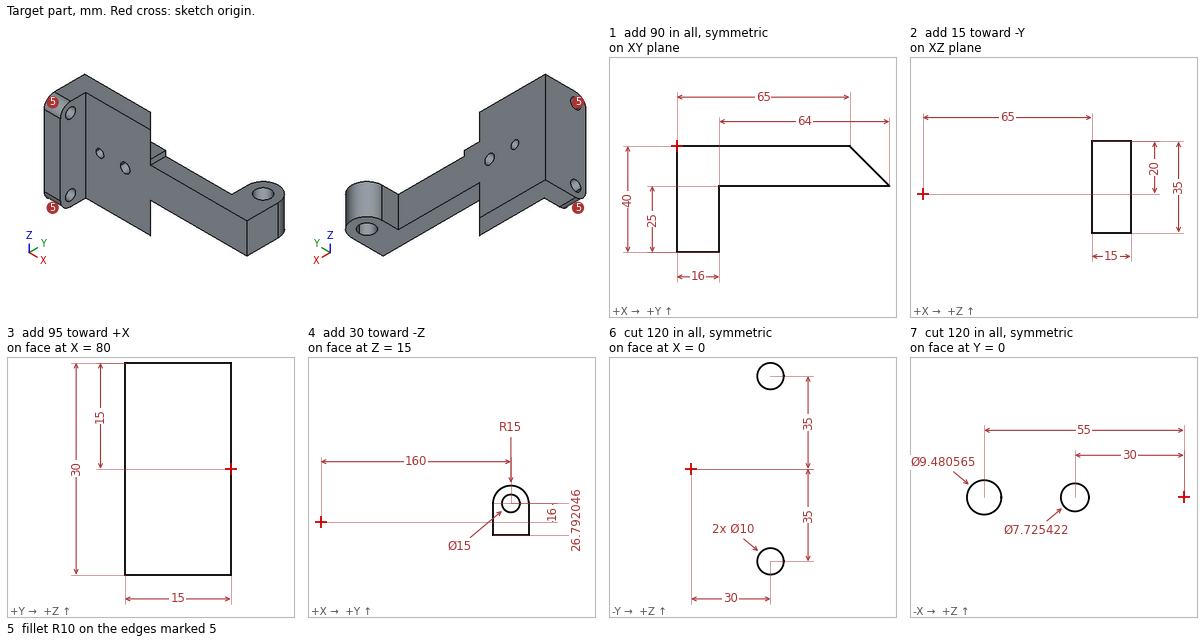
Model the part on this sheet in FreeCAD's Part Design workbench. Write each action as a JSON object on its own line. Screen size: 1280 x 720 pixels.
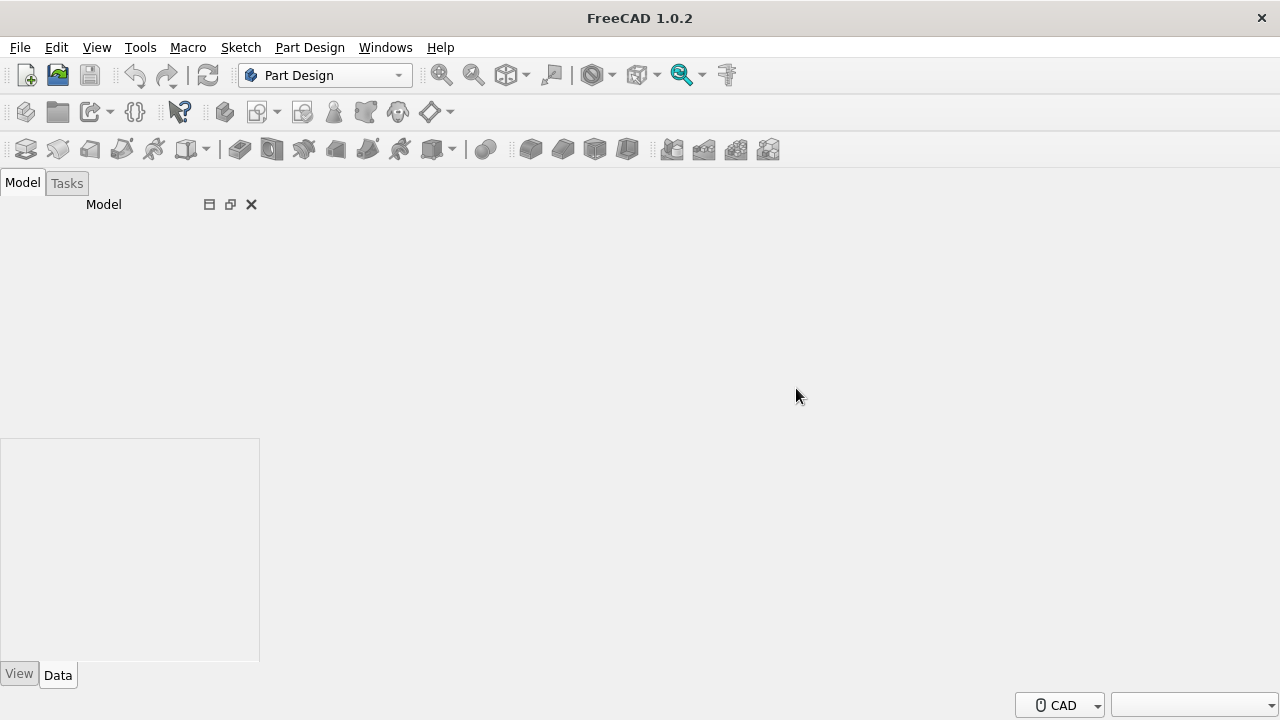
{"action": "left_click", "coordinate": [26, 76]}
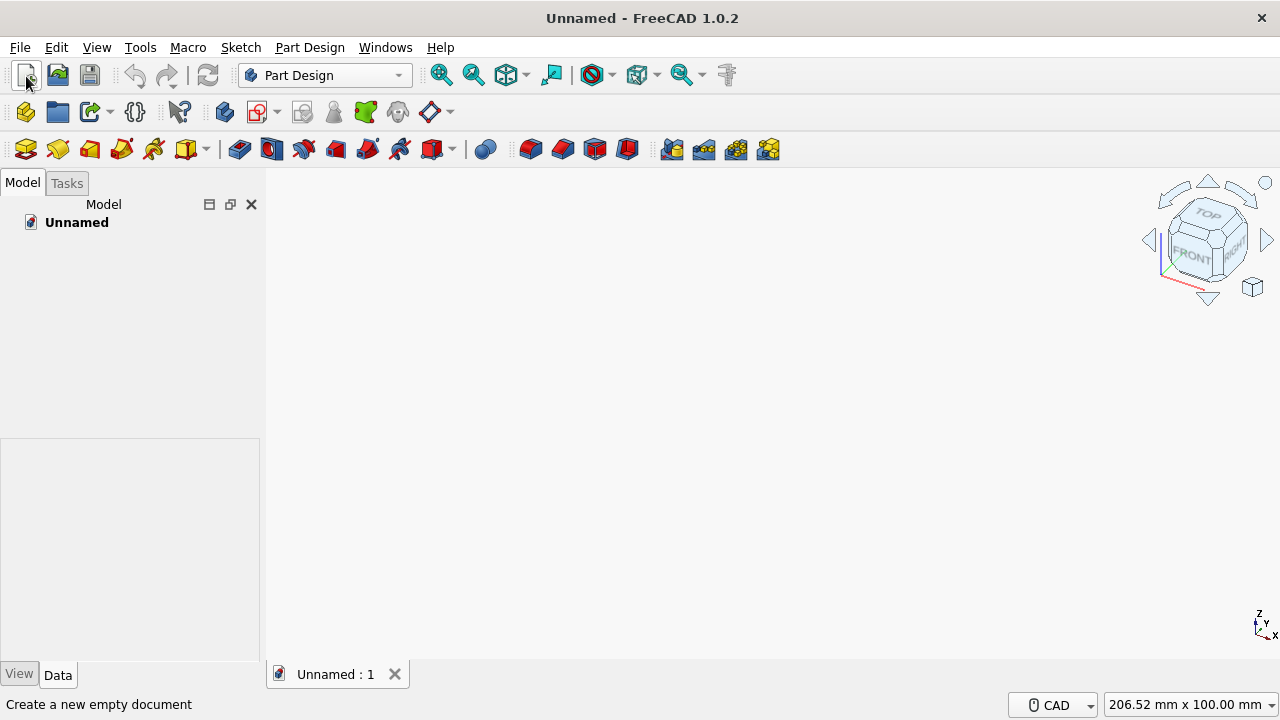
{"action": "left_click", "coordinate": [258, 112]}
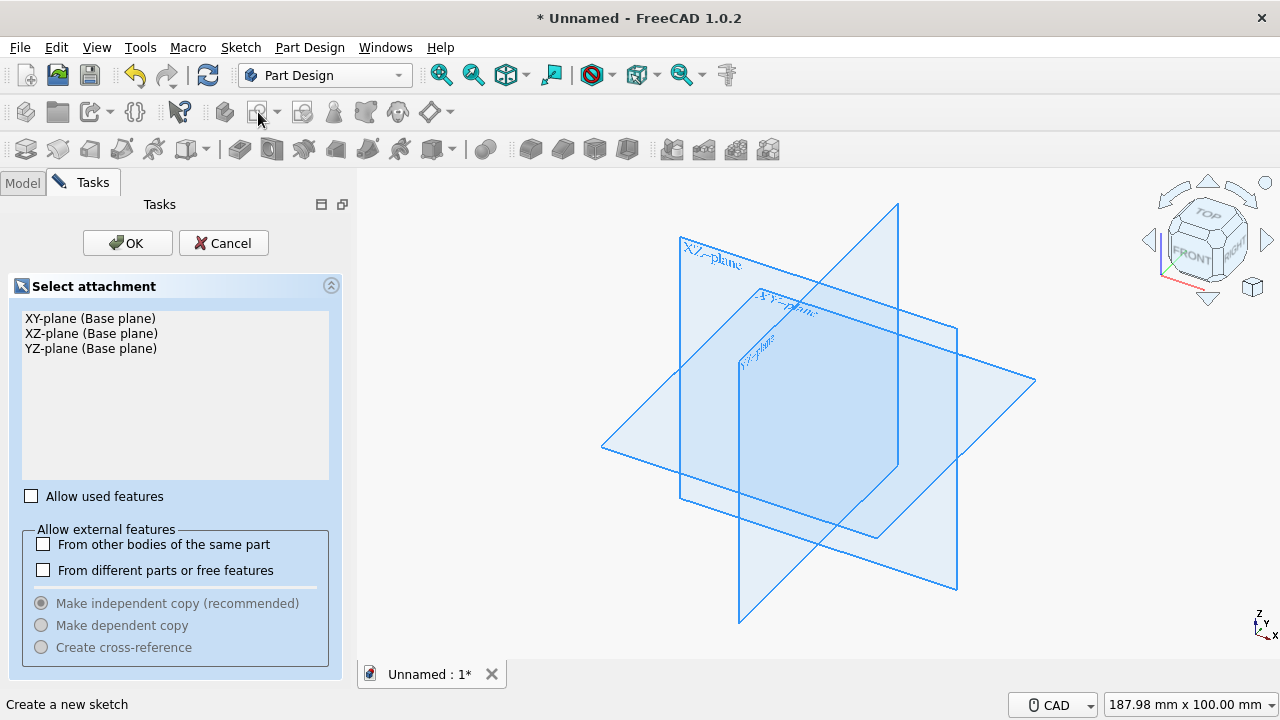
{"action": "left_click", "coordinate": [82, 318]}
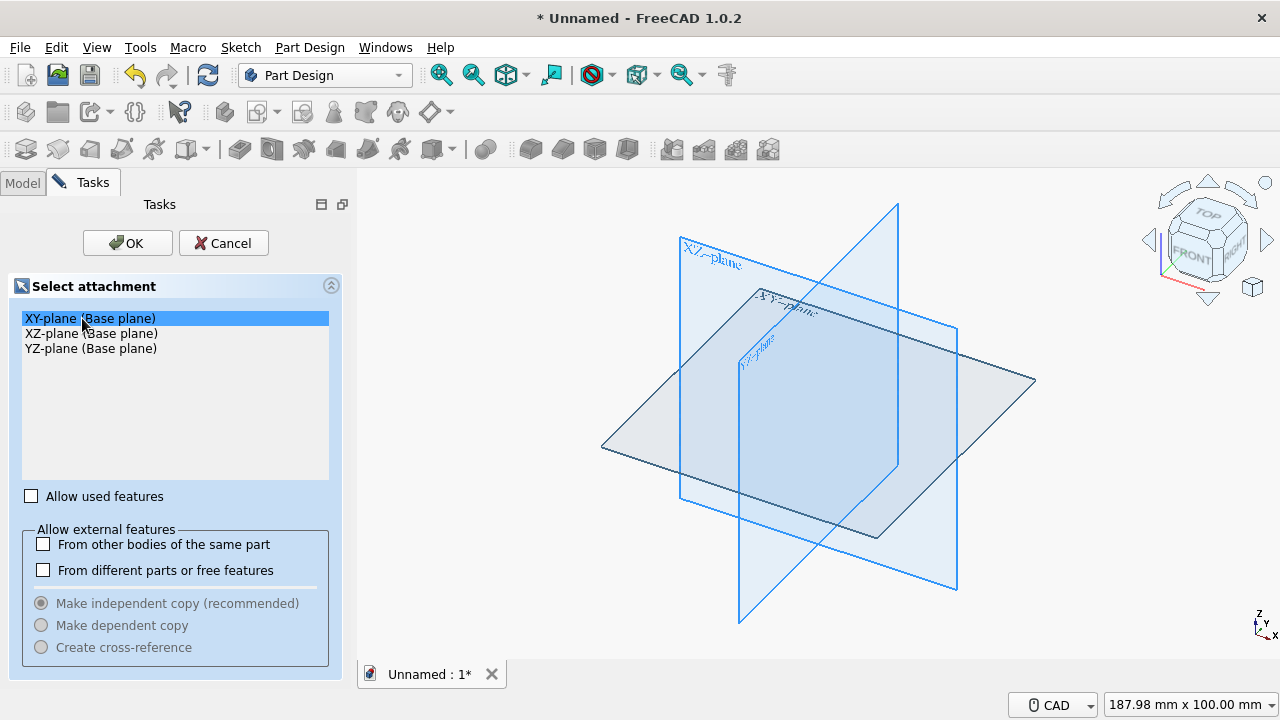
{"action": "left_click", "coordinate": [128, 243]}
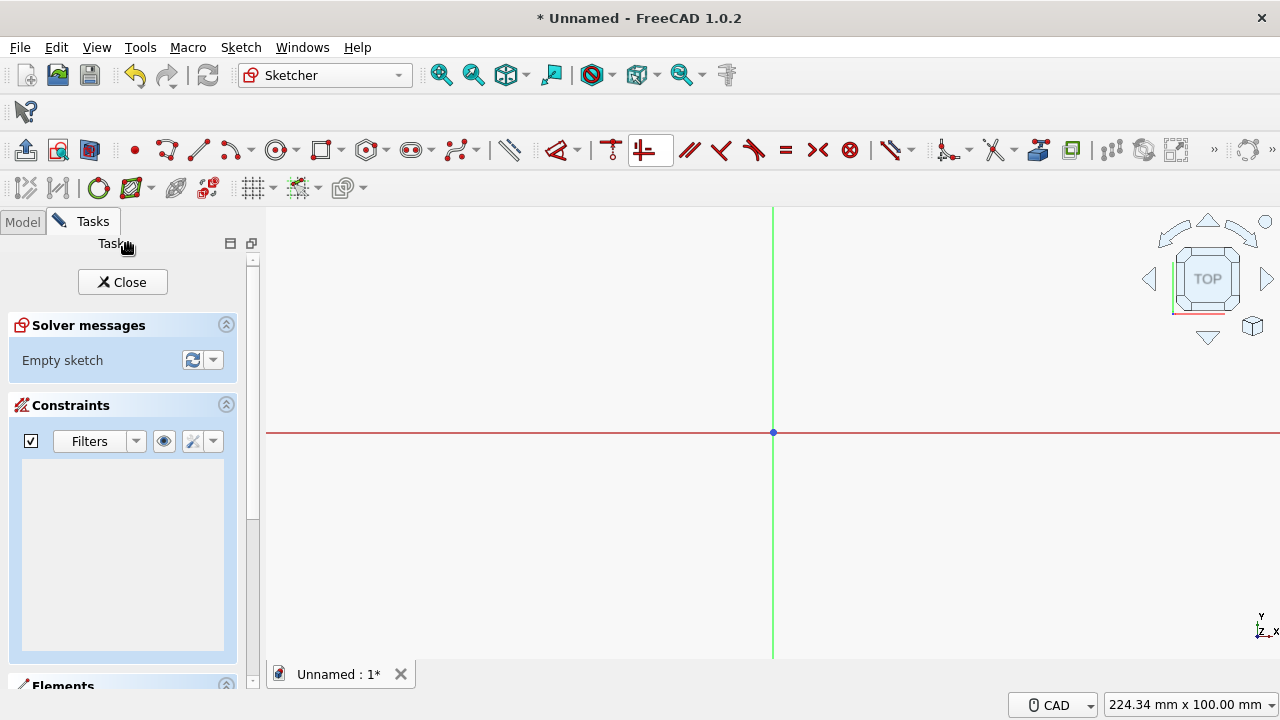
{"action": "scroll", "coordinate": [294, 235], "scroll_direction": "down", "scroll_amount": 1}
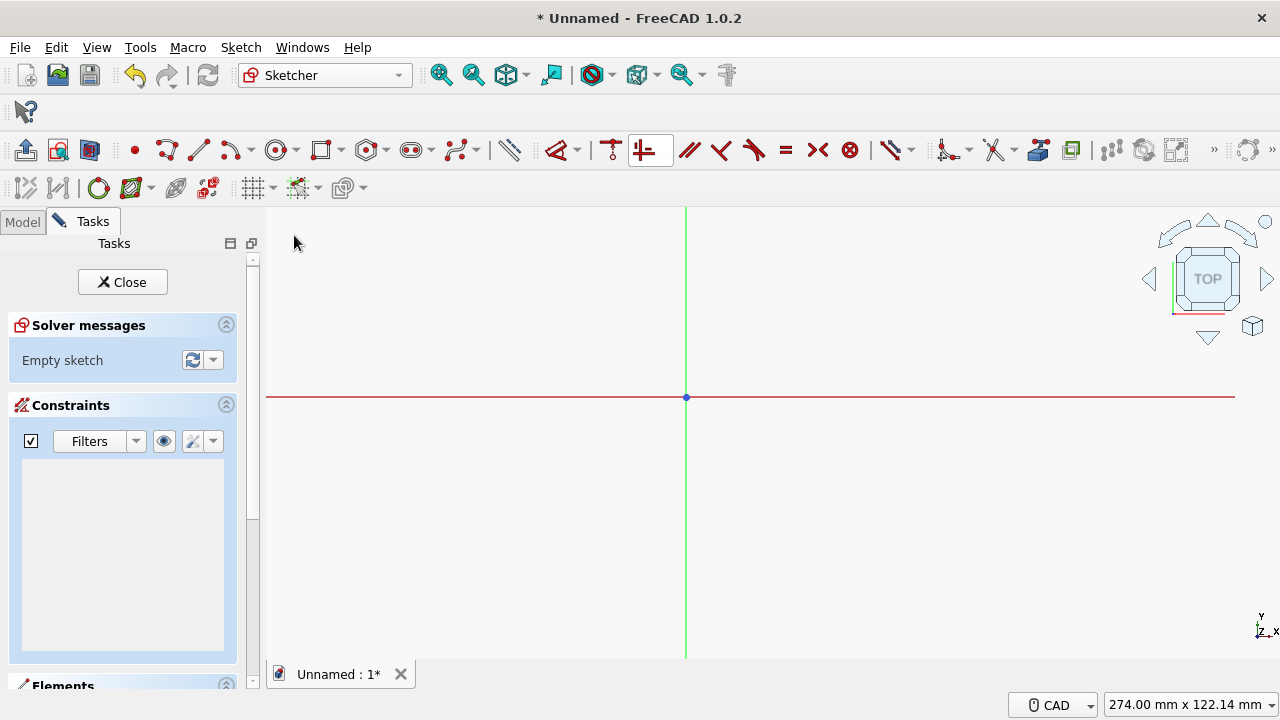
{"action": "scroll", "coordinate": [992, 518], "scroll_direction": "up", "scroll_amount": 3}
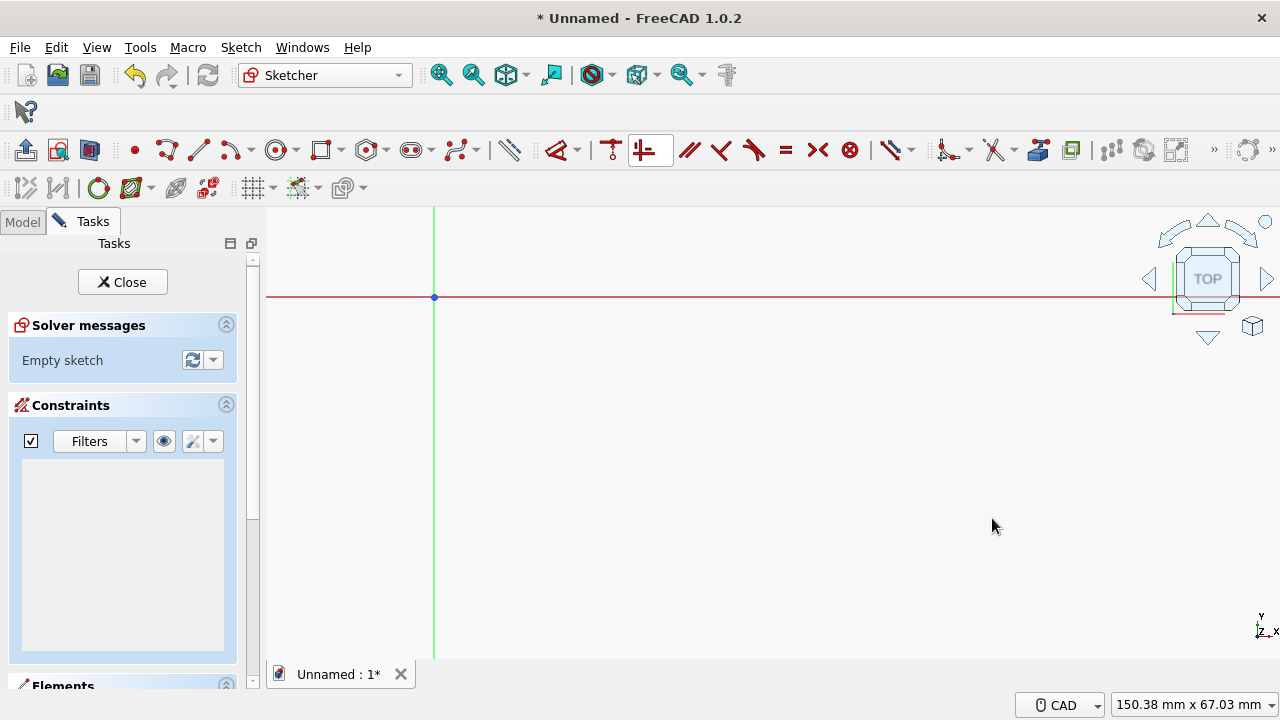
{"action": "left_click", "coordinate": [168, 150]}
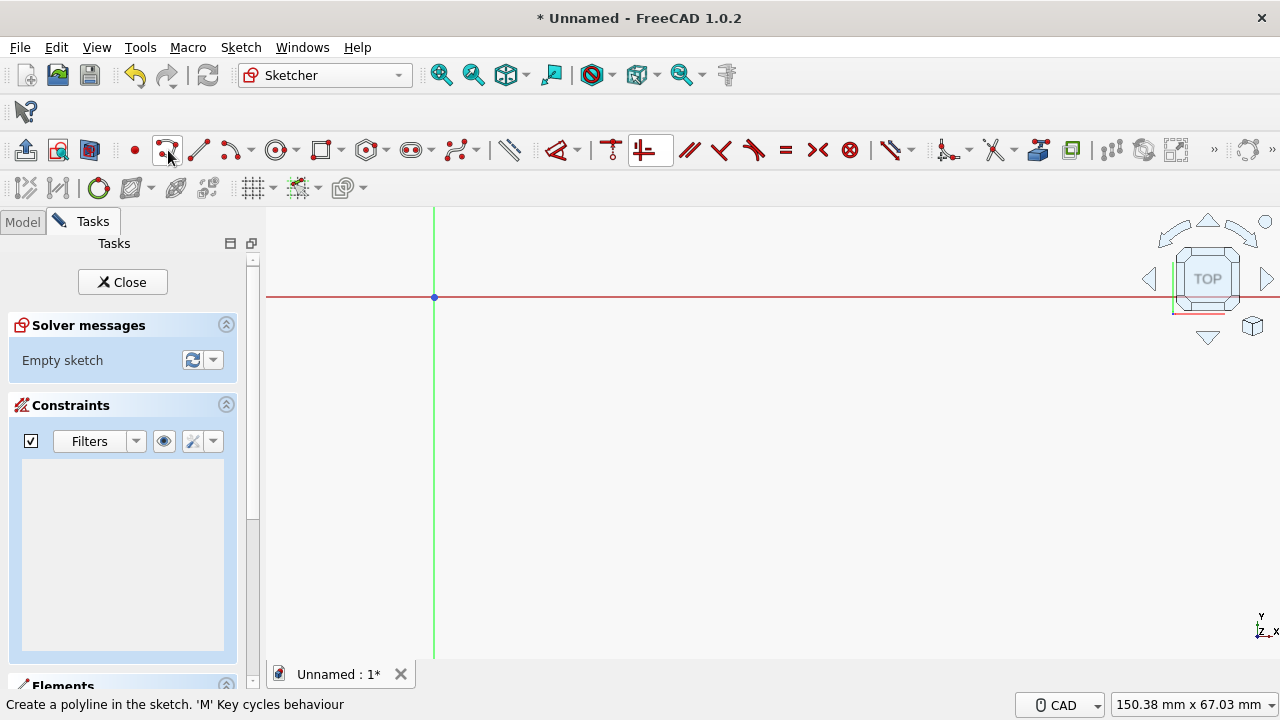
{"action": "left_click", "coordinate": [434, 297]}
{"action": "left_click", "coordinate": [443, 567]}
{"action": "left_click", "coordinate": [542, 567]}
{"action": "left_click", "coordinate": [542, 398]}
{"action": "left_click", "coordinate": [974, 398]}
{"action": "left_click", "coordinate": [872, 306]}
{"action": "left_click", "coordinate": [434, 297]}
{"action": "key", "text": "Escape"}
{"action": "key", "text": "Escape"}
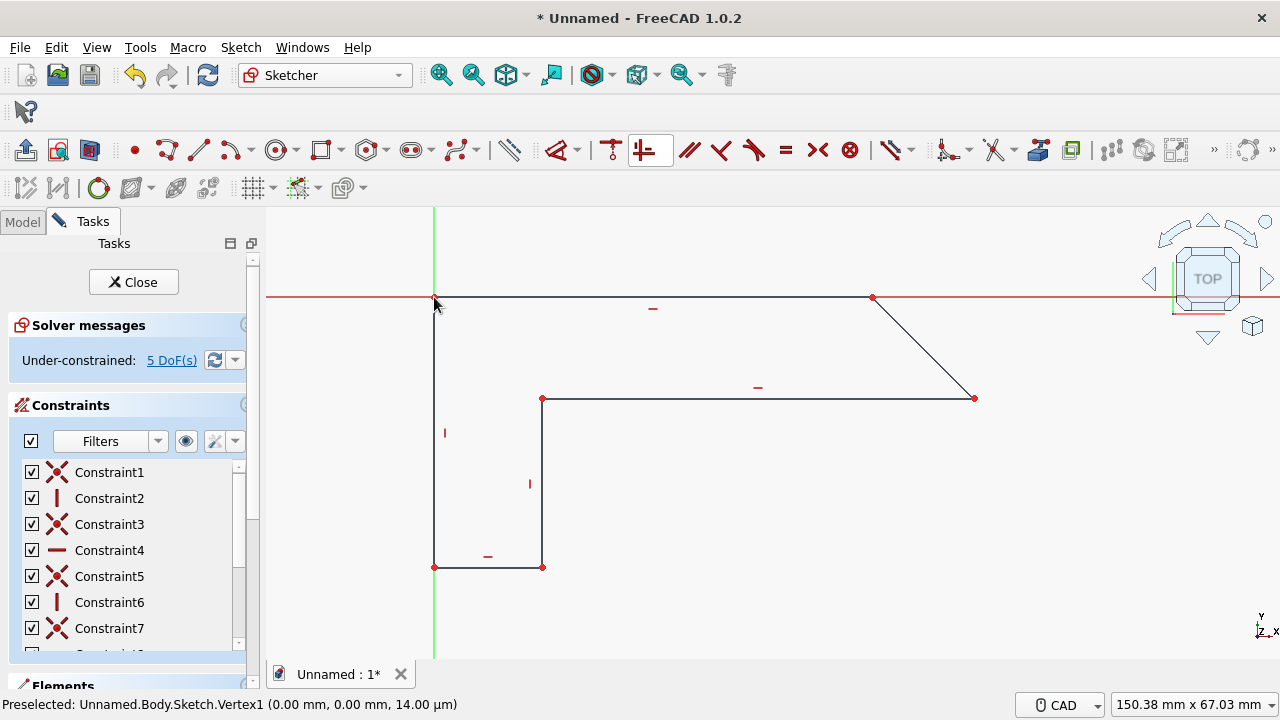
{"action": "left_click", "coordinate": [556, 150]}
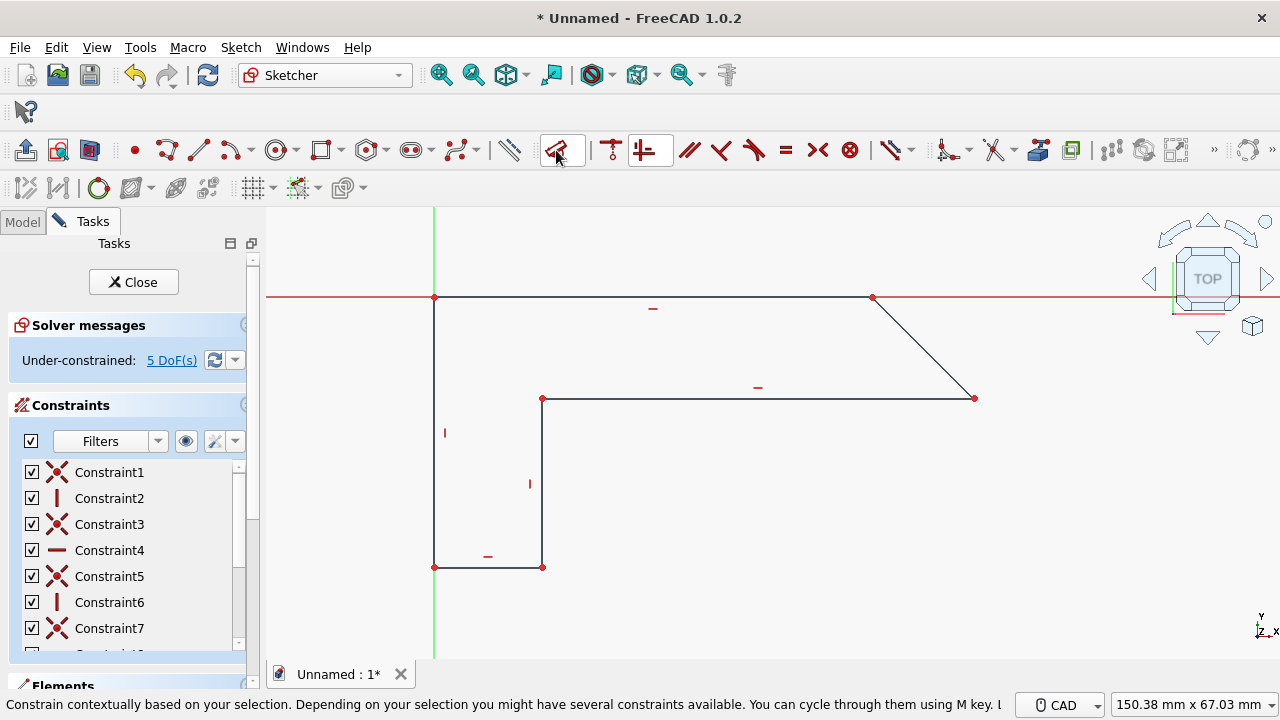
{"action": "left_click", "coordinate": [434, 378]}
{"action": "left_click", "coordinate": [400, 433]}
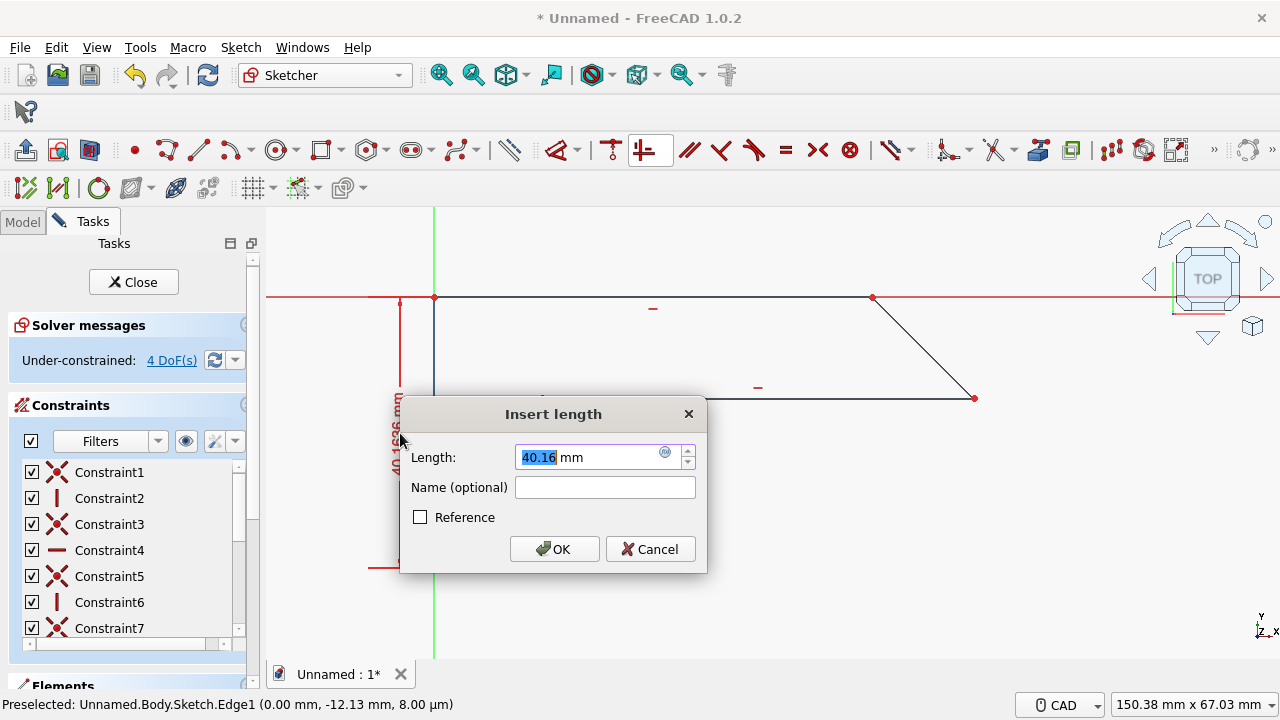
{"action": "type", "text": "40"}
{"action": "key", "text": "Return"}